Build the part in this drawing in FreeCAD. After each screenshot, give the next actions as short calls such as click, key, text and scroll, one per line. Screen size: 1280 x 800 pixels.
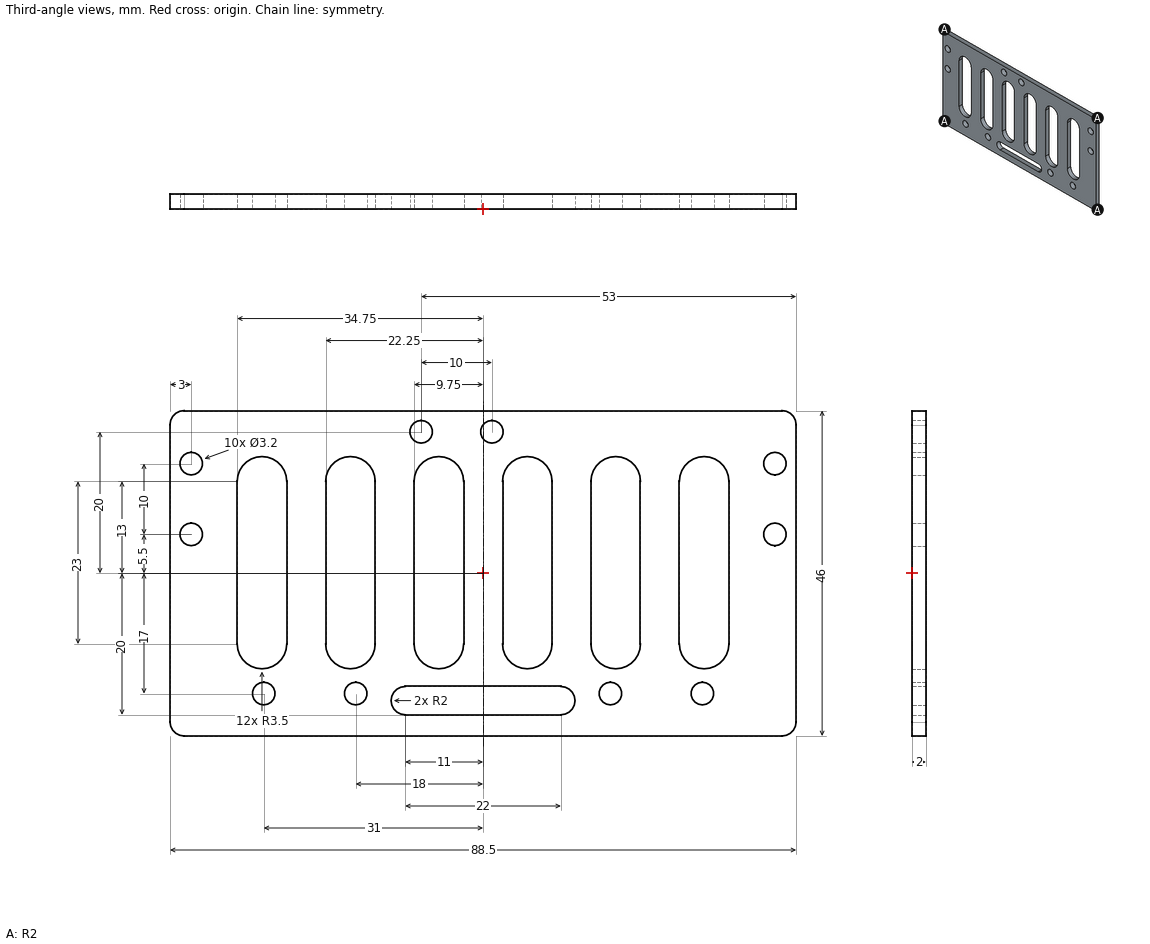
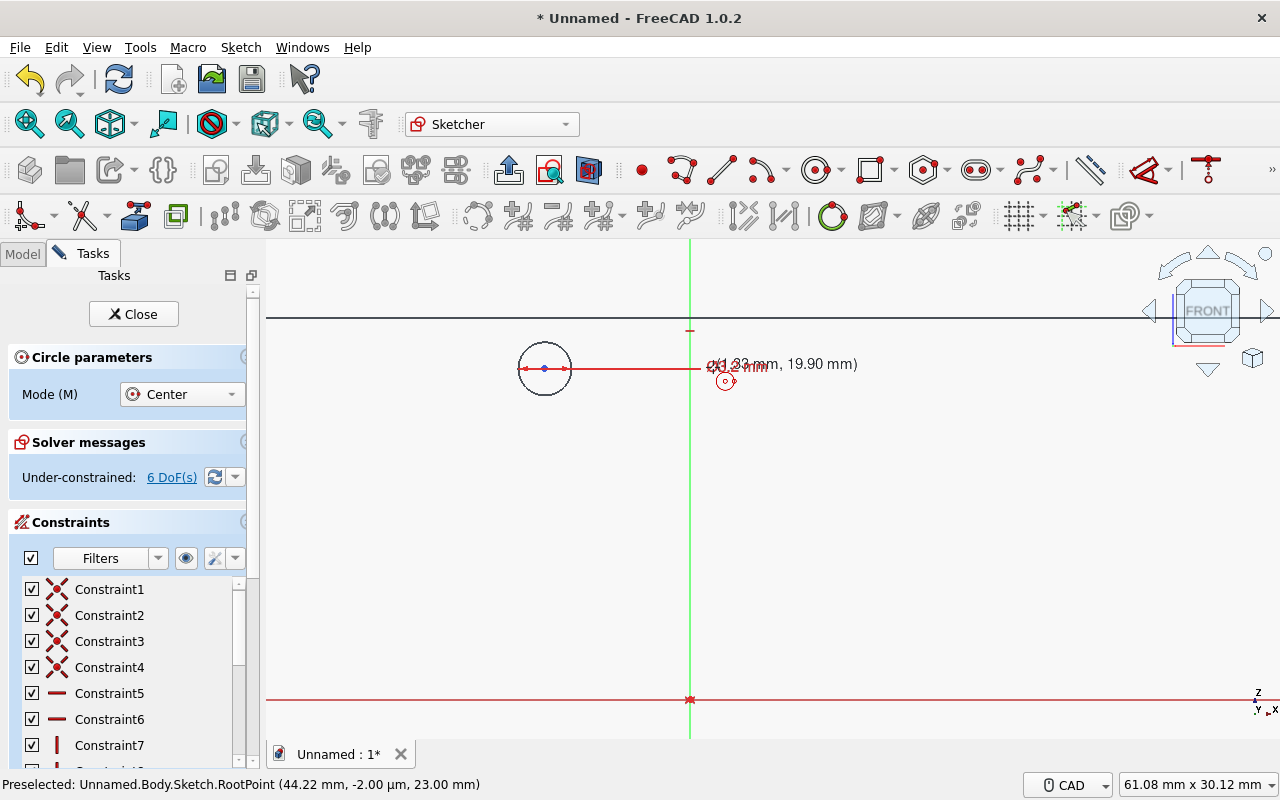
click(711, 368)
move(730, 349)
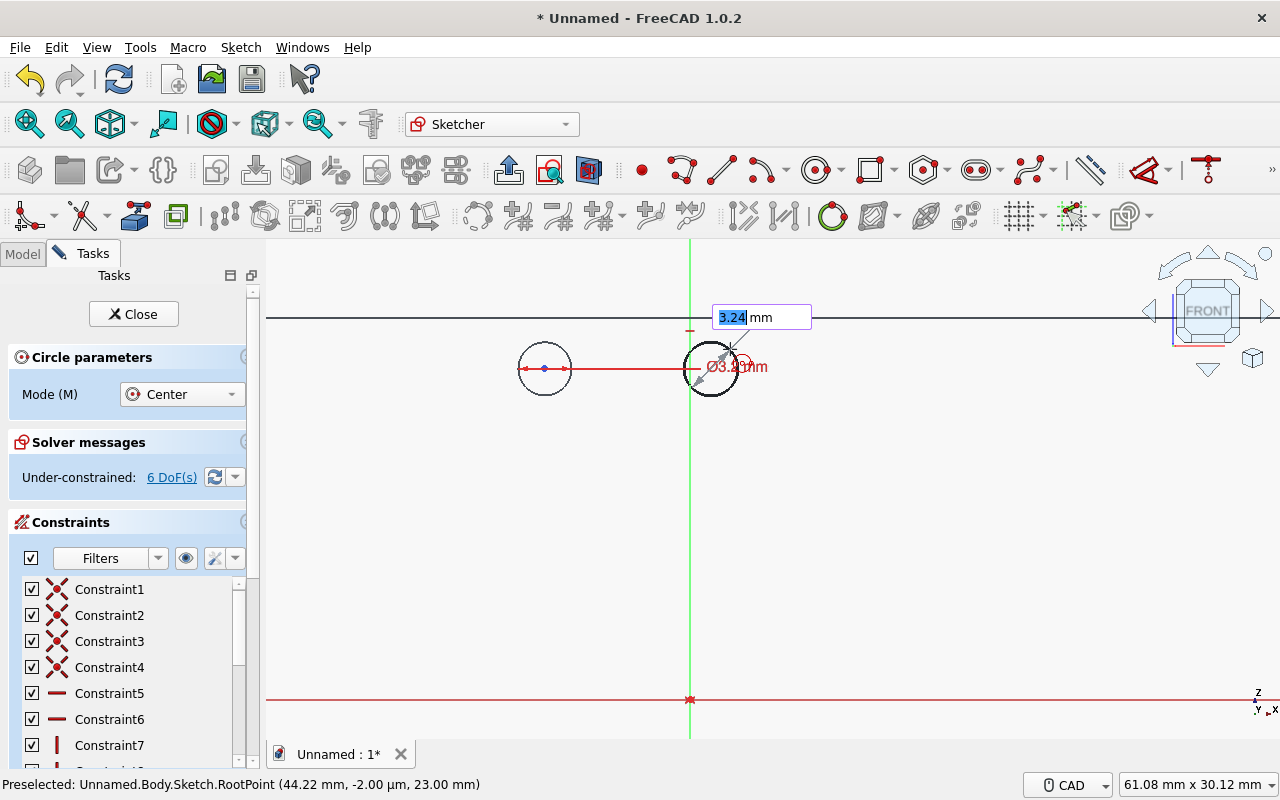
text(3.2)
key(Return)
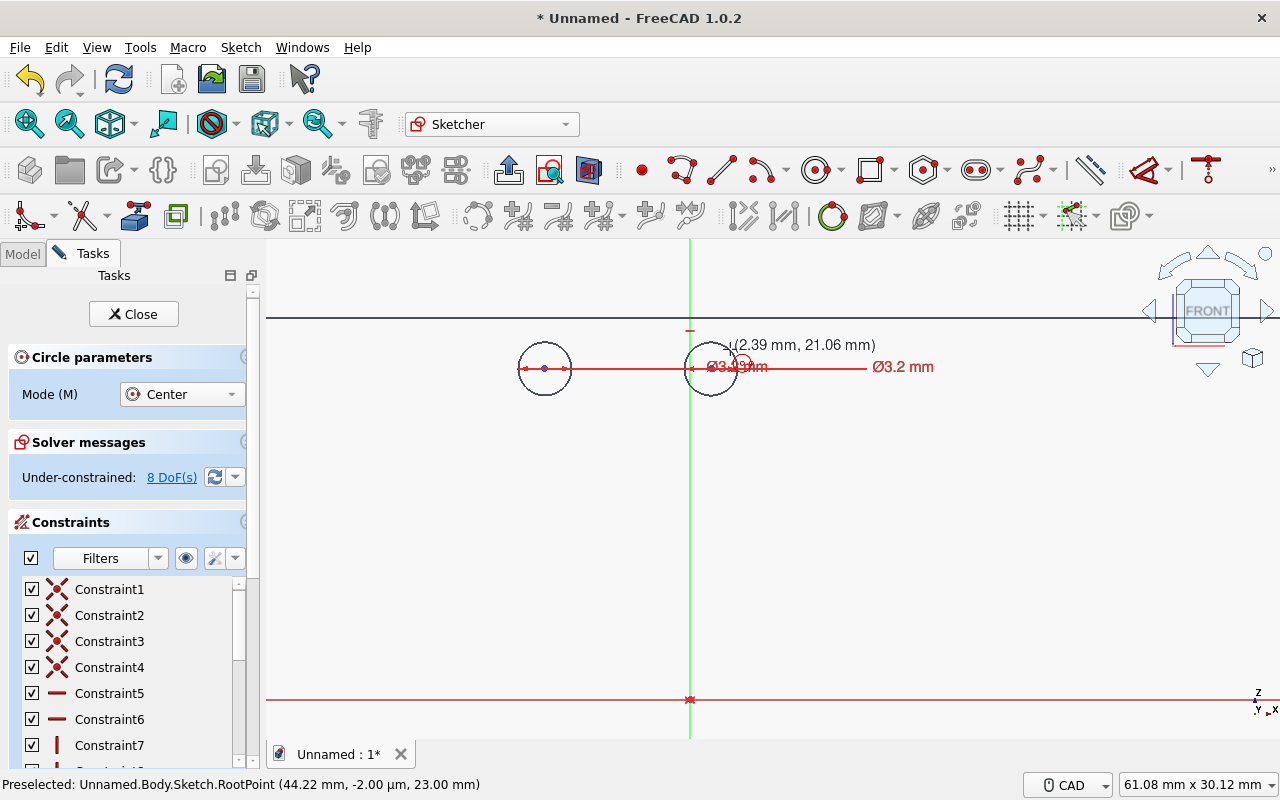
scroll(713, 366, down, 5)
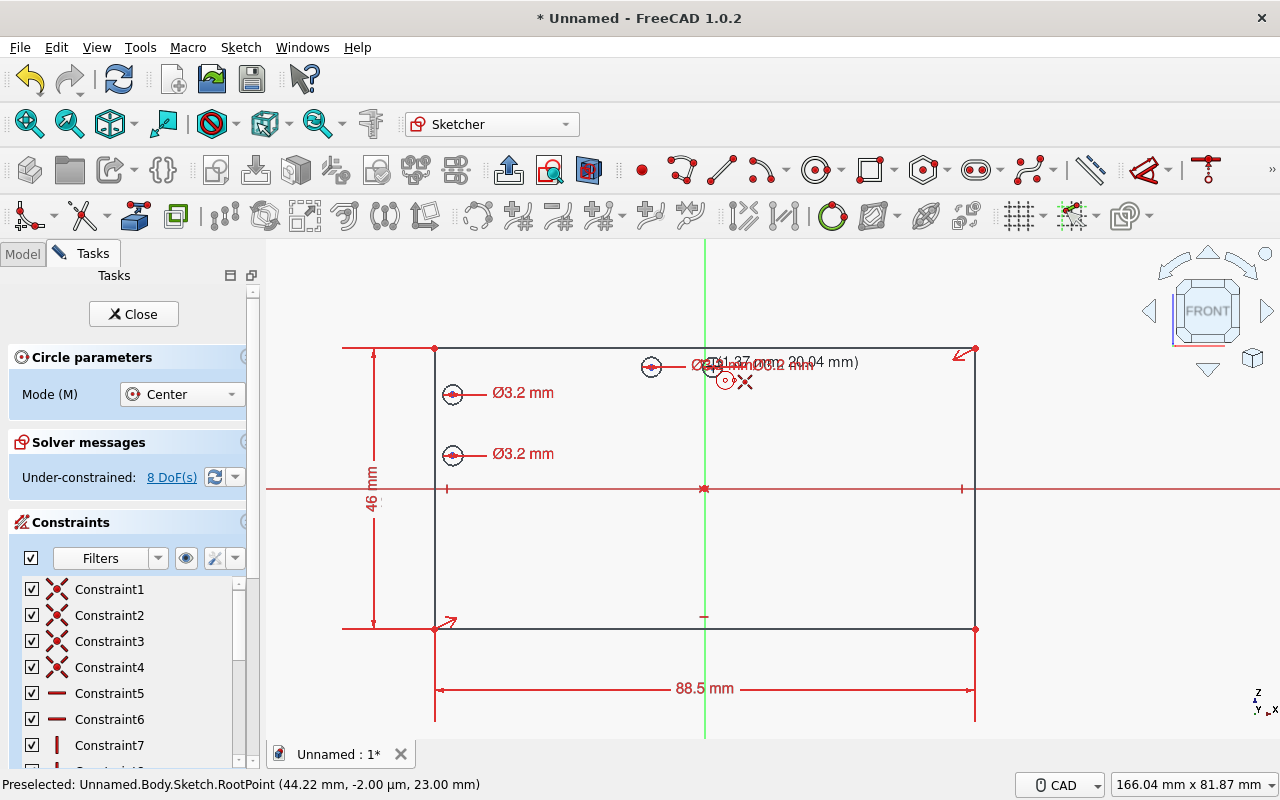
scroll(957, 394, up, 5)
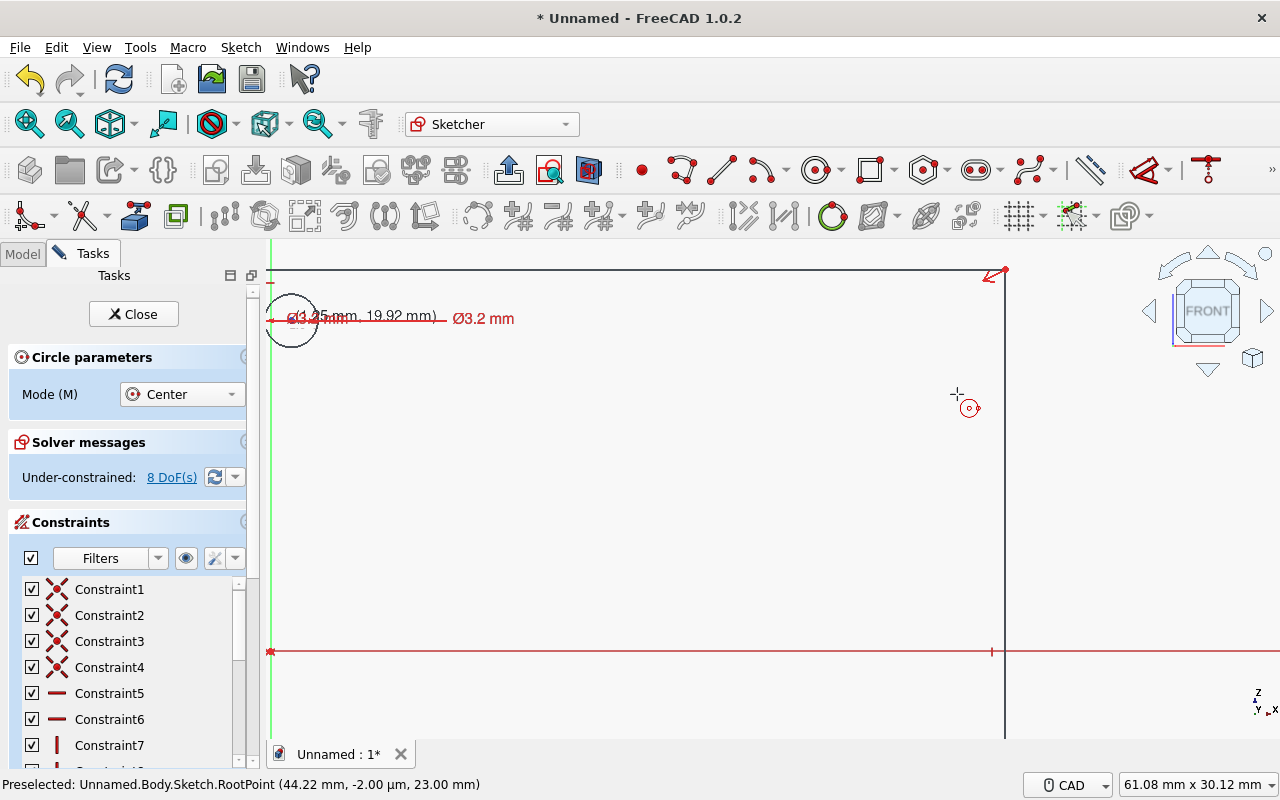
click(955, 394)
move(974, 375)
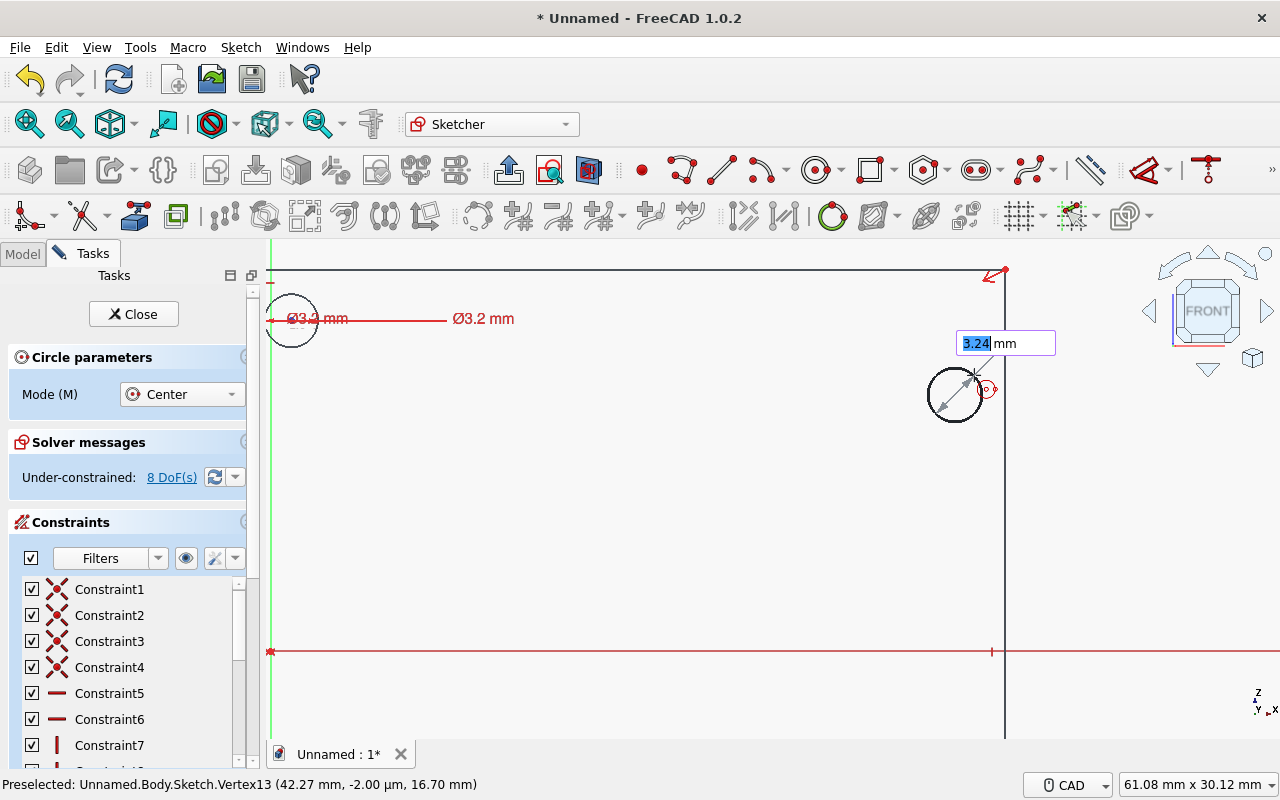
text(3.2)
key(Return)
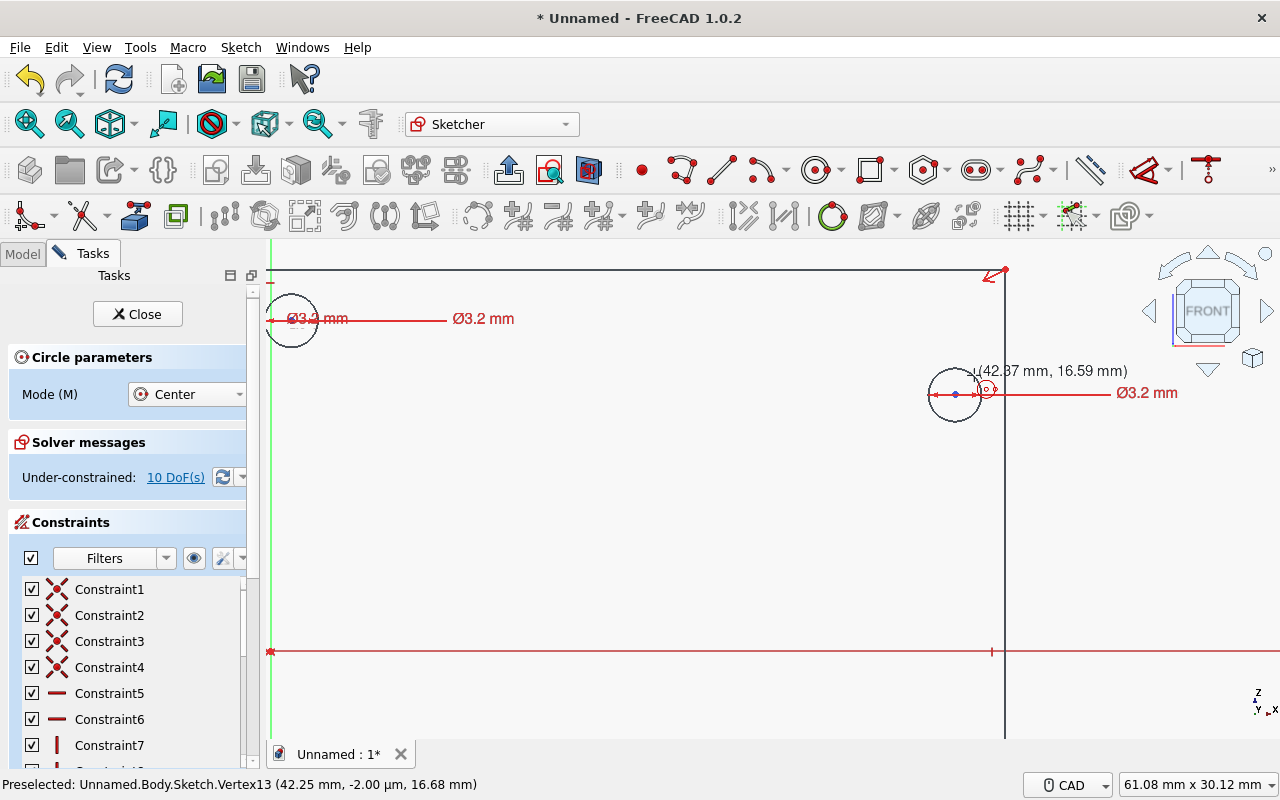
click(955, 560)
move(974, 541)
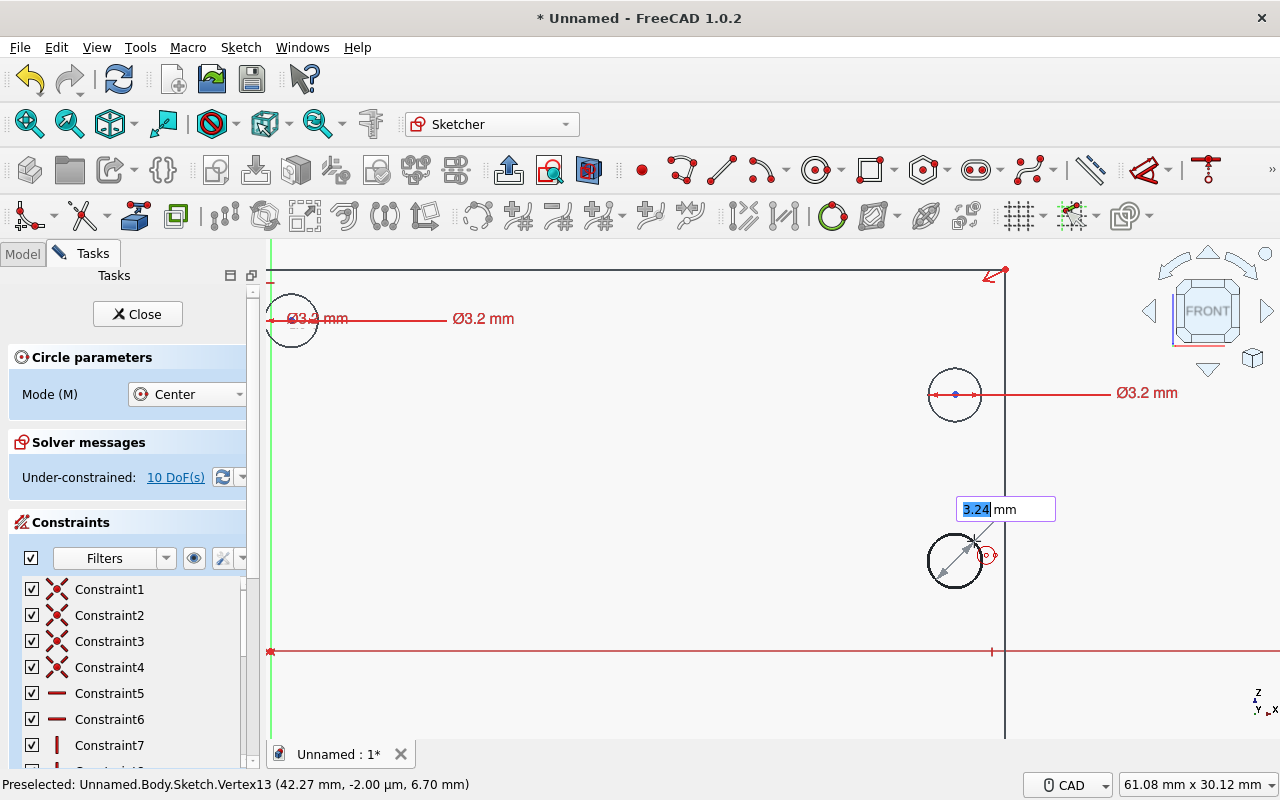
text(3.2)
key(Return)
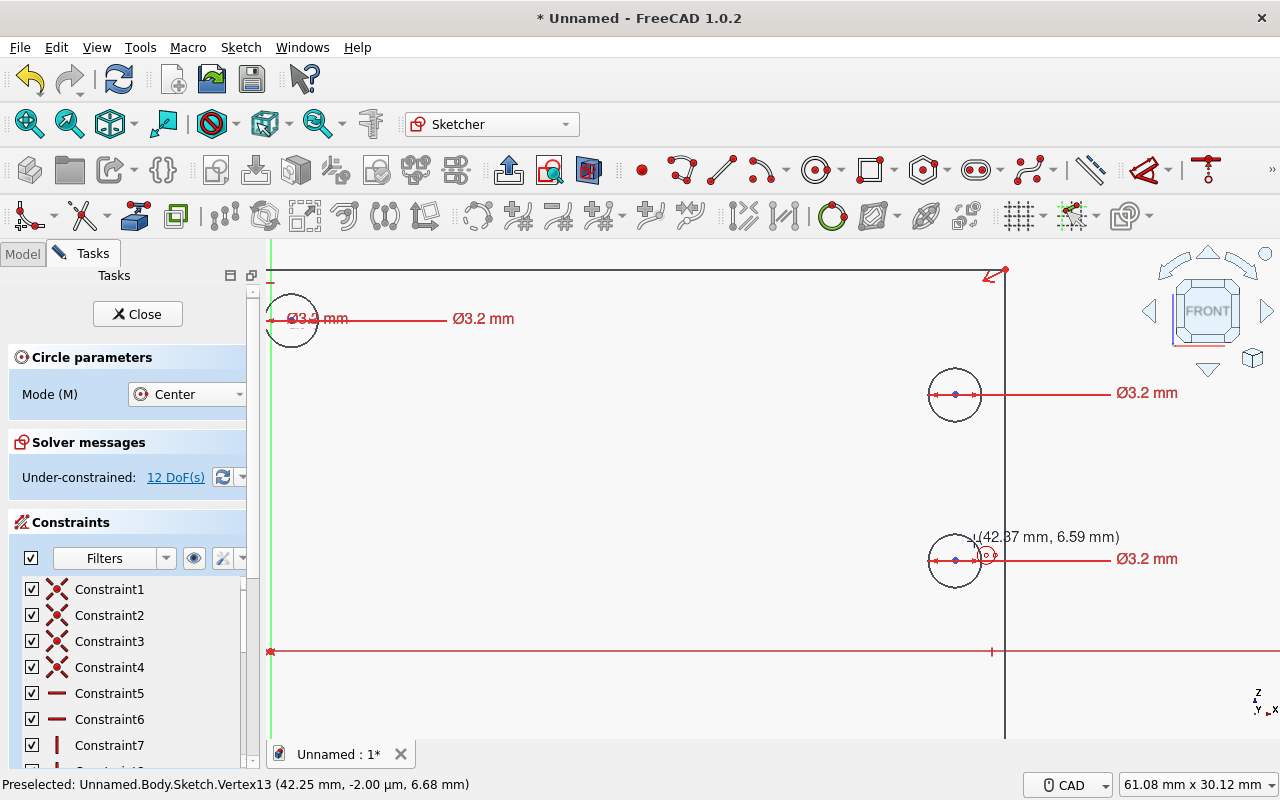
scroll(957, 394, down, 5)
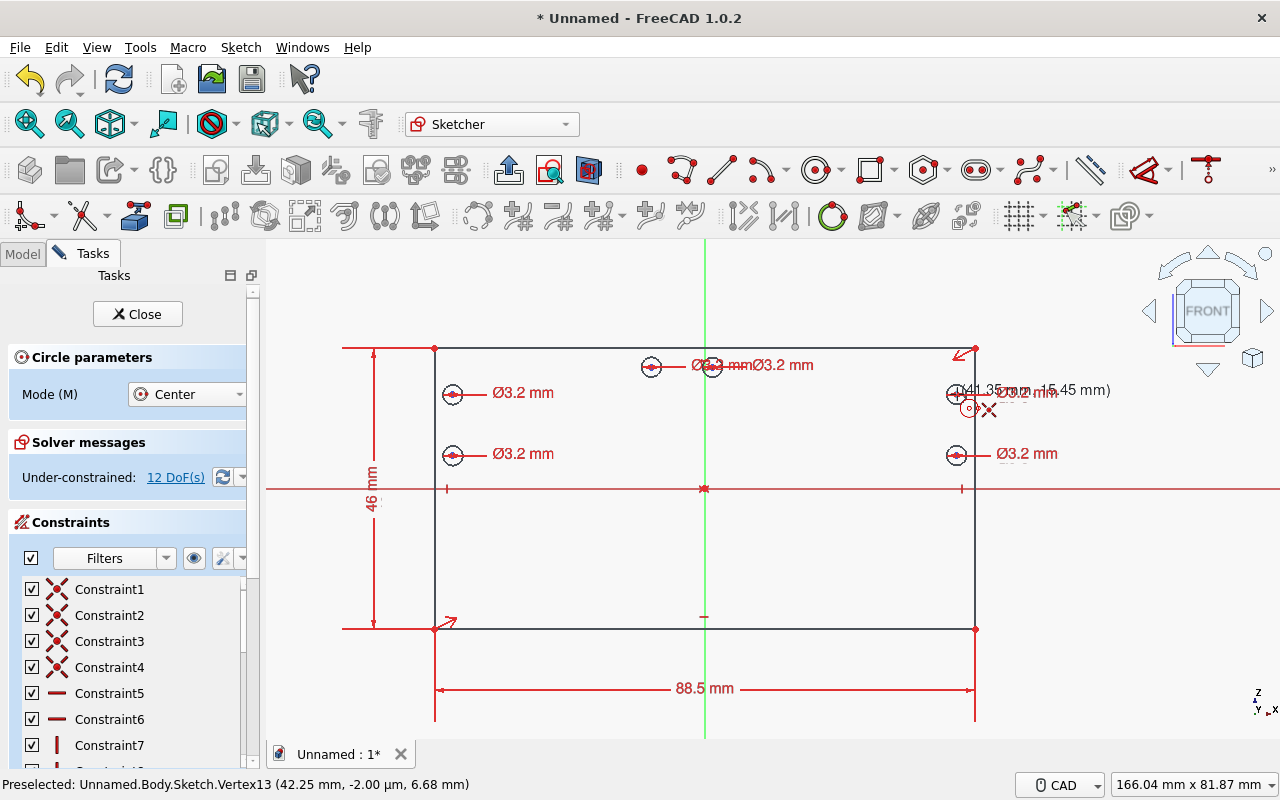
scroll(516, 593, up, 5)